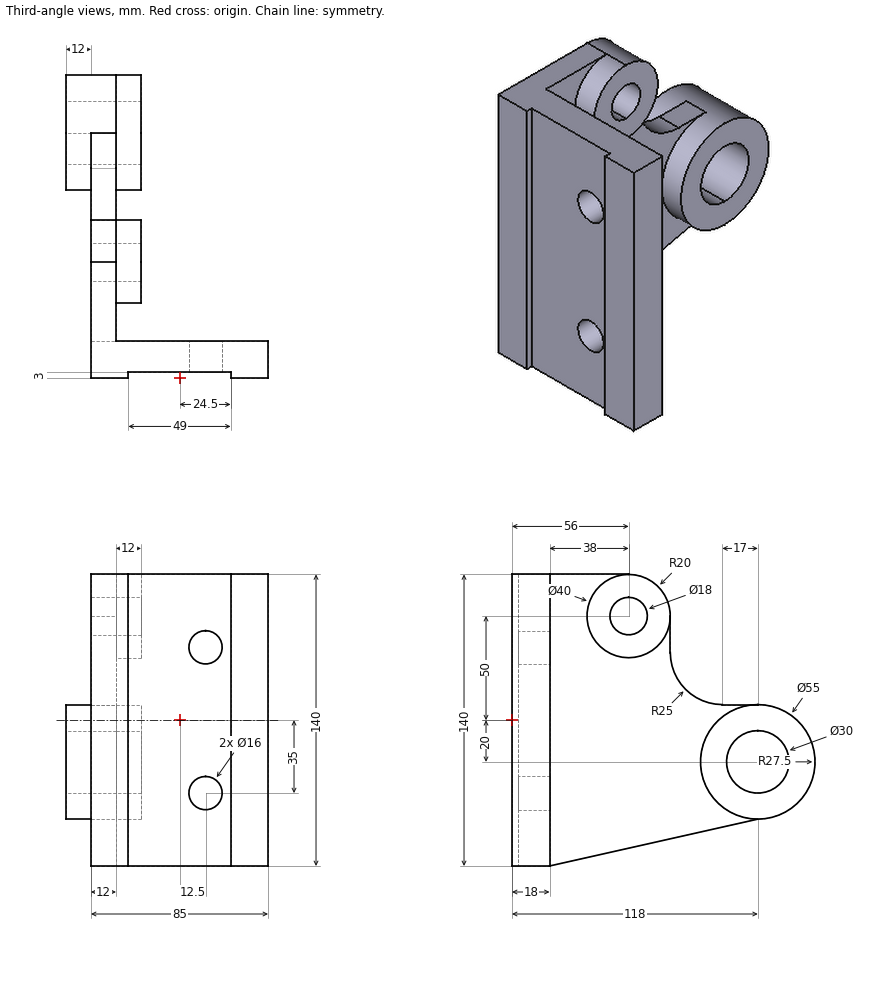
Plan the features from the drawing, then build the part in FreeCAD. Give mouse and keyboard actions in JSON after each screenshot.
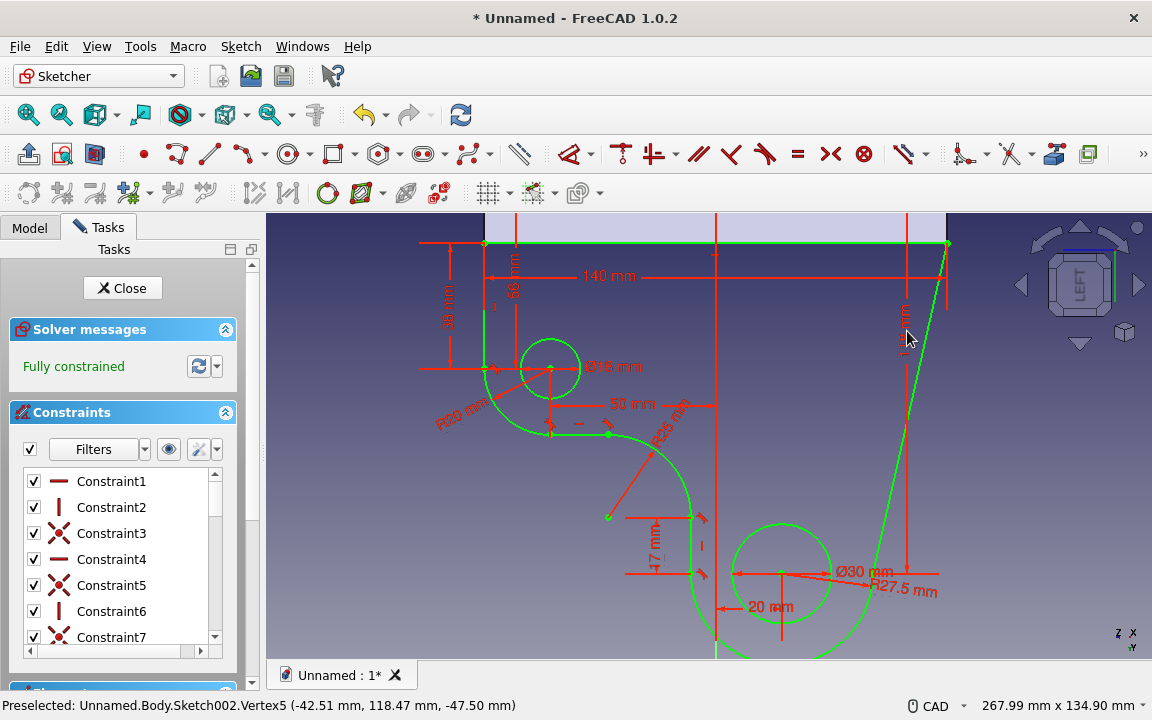
{"action": "left_click", "coordinate": [123, 288]}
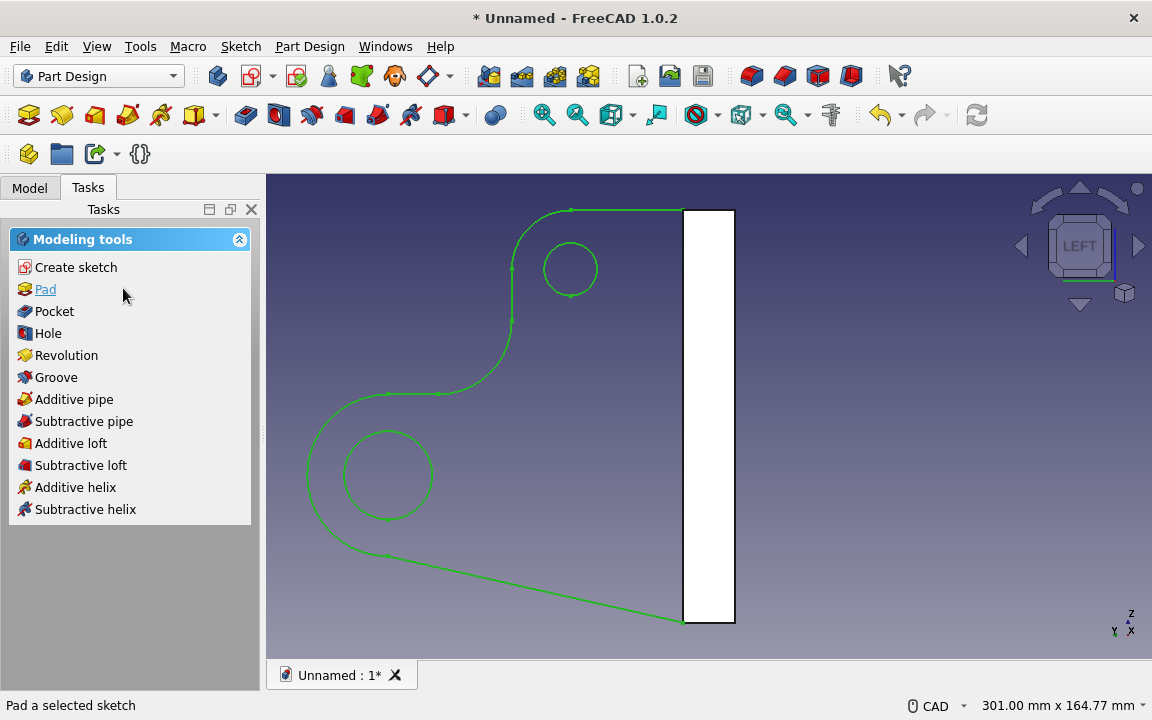
{"action": "left_click", "coordinate": [29, 116]}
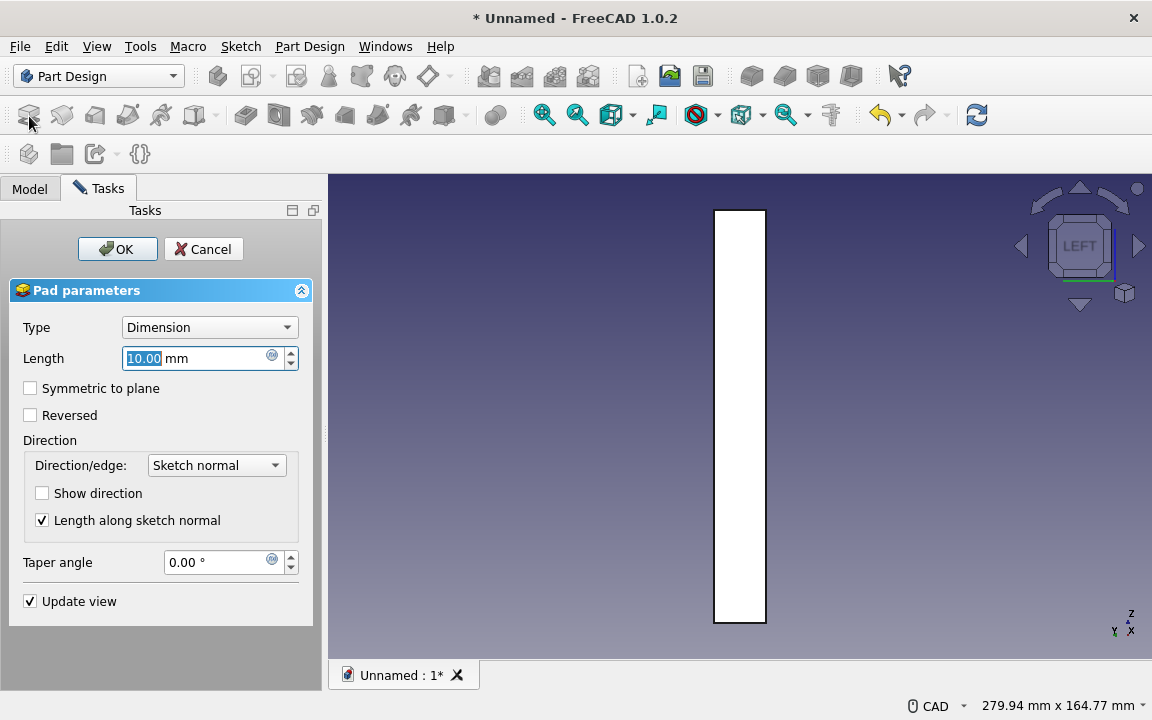
{"action": "type", "text": "12"}
{"action": "key", "text": "Tab"}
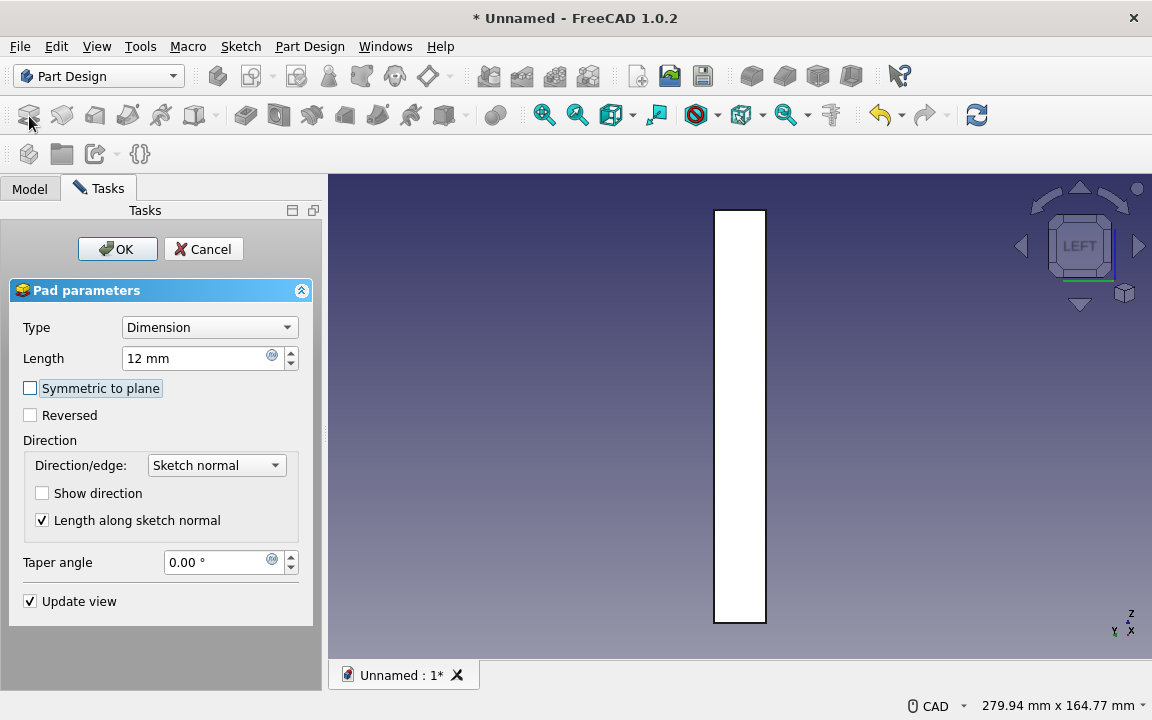
{"action": "left_click", "coordinate": [31, 415]}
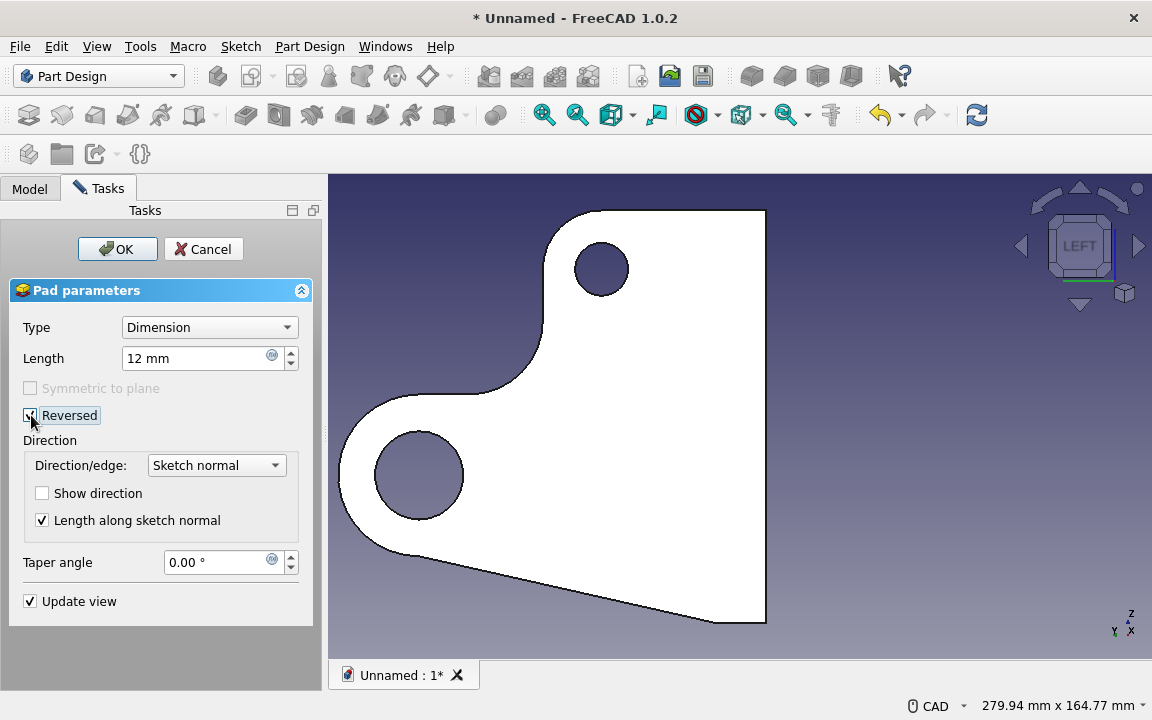
{"action": "left_click", "coordinate": [118, 249]}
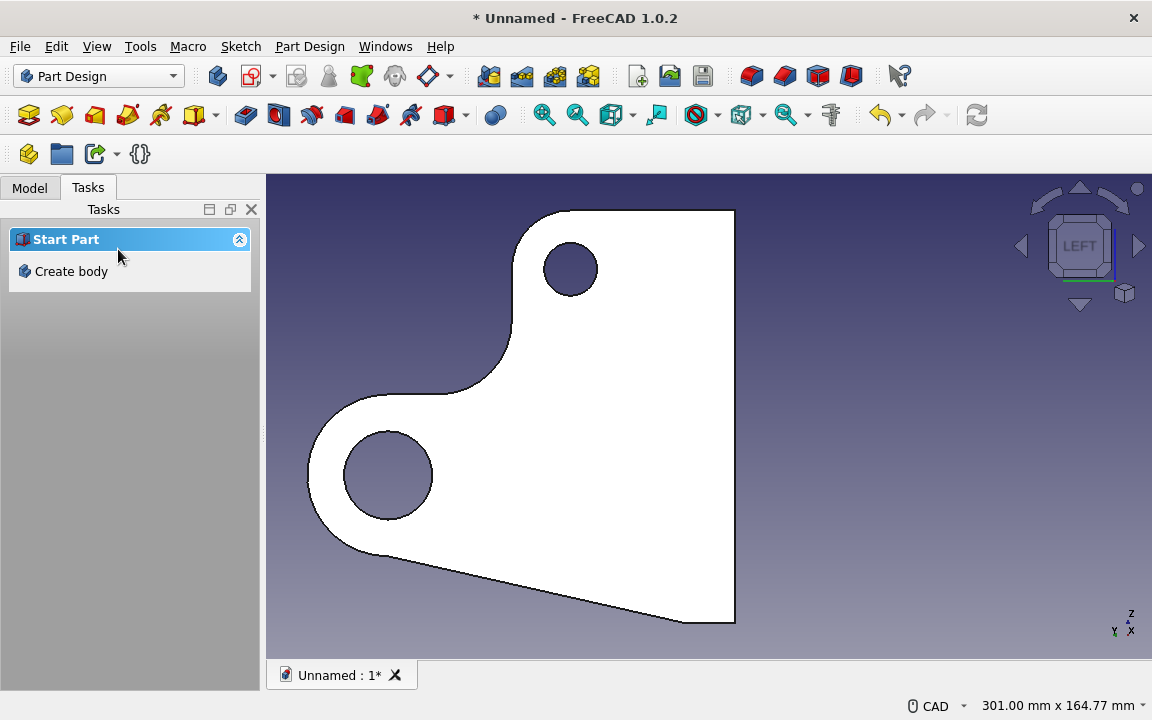
{"action": "key", "text": "0"}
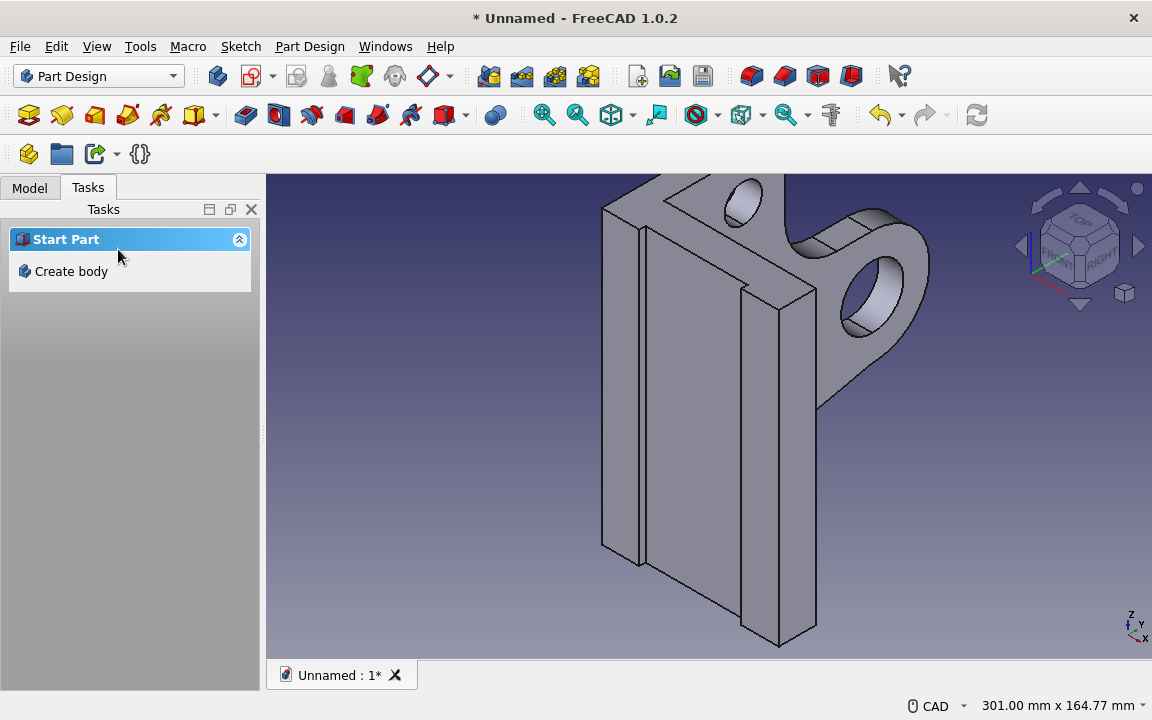
{"action": "key", "text": "v f"}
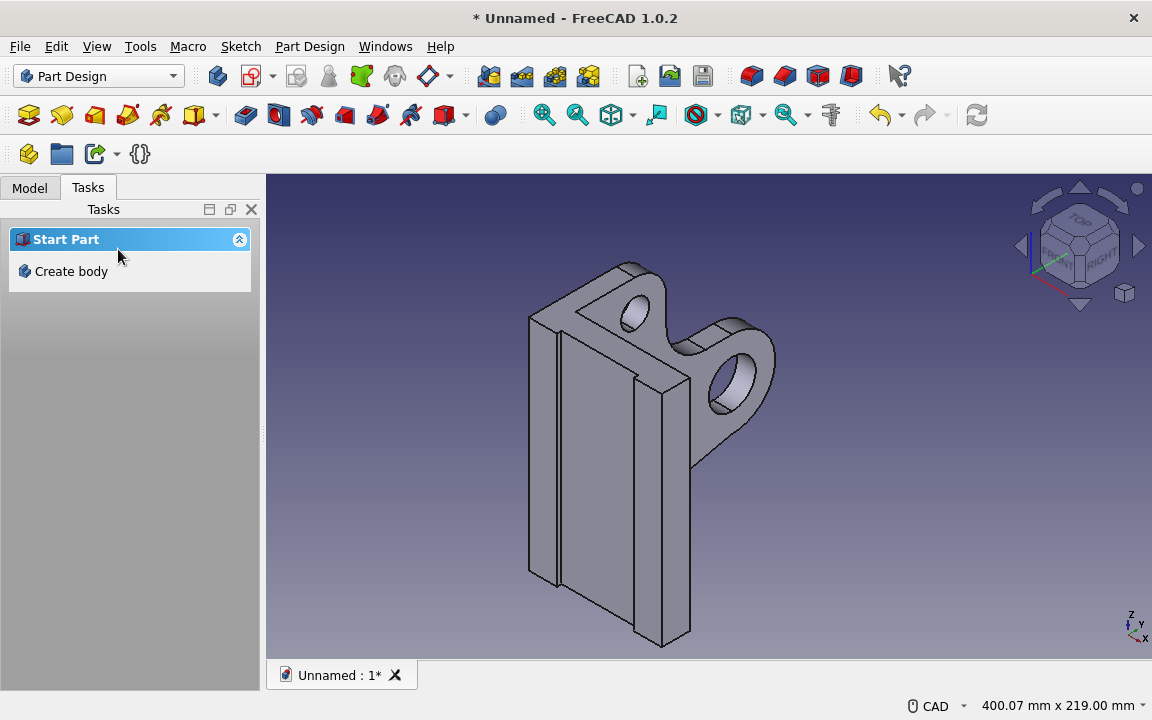
{"action": "key", "text": "3"}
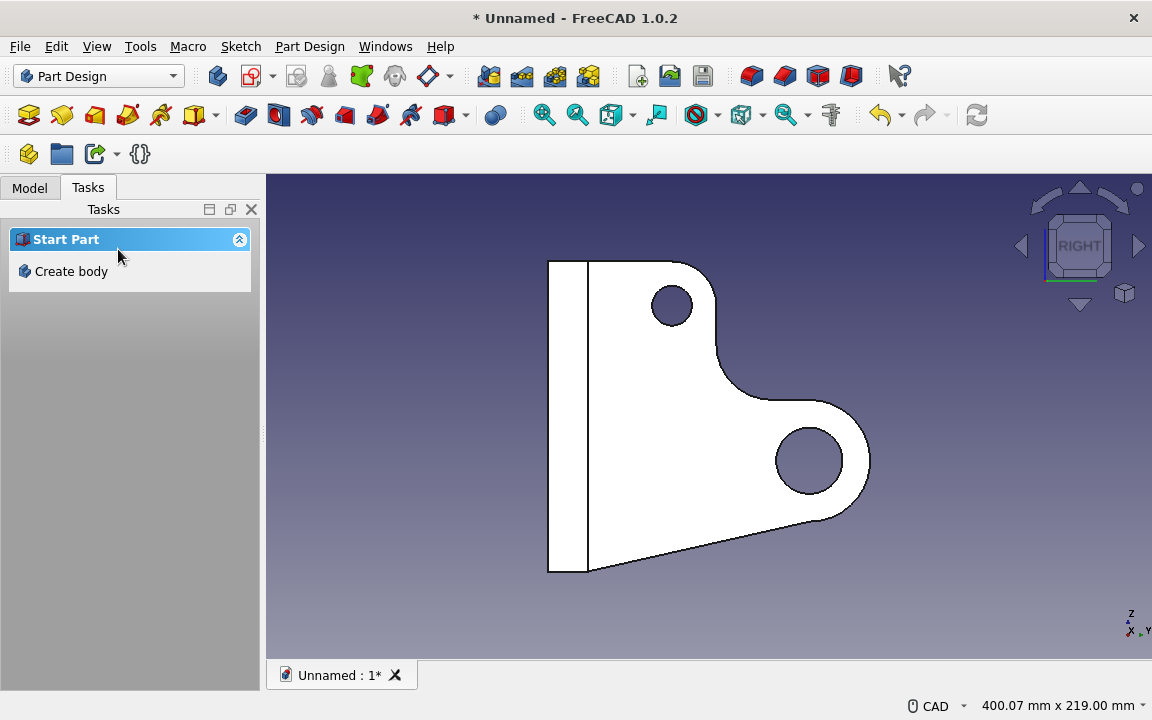
{"action": "left_click", "coordinate": [689, 460]}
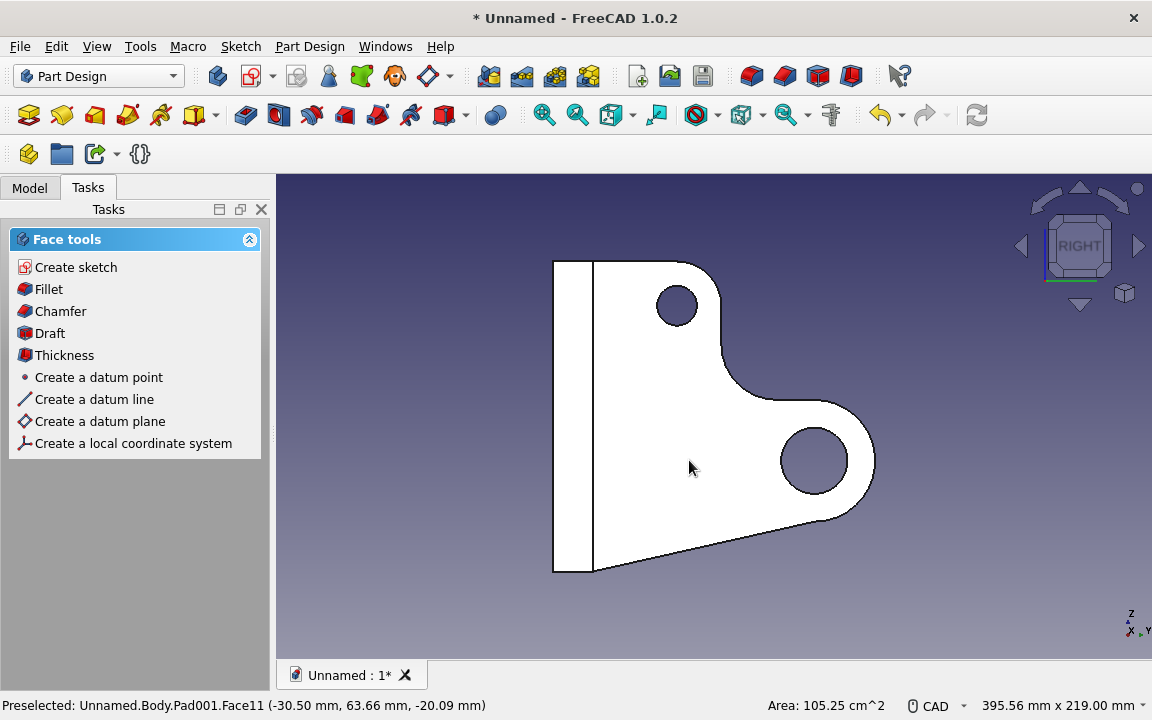
{"action": "left_click", "coordinate": [250, 76]}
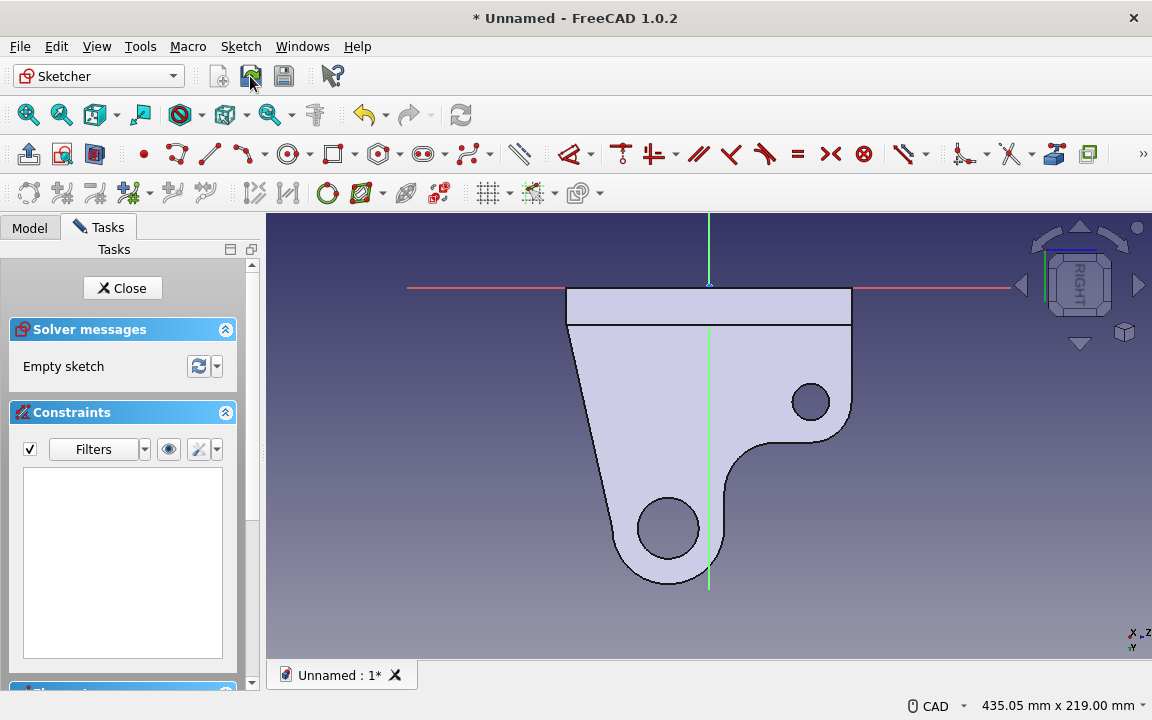
{"action": "scroll", "coordinate": [950, 279], "scroll_direction": "up", "scroll_amount": 3}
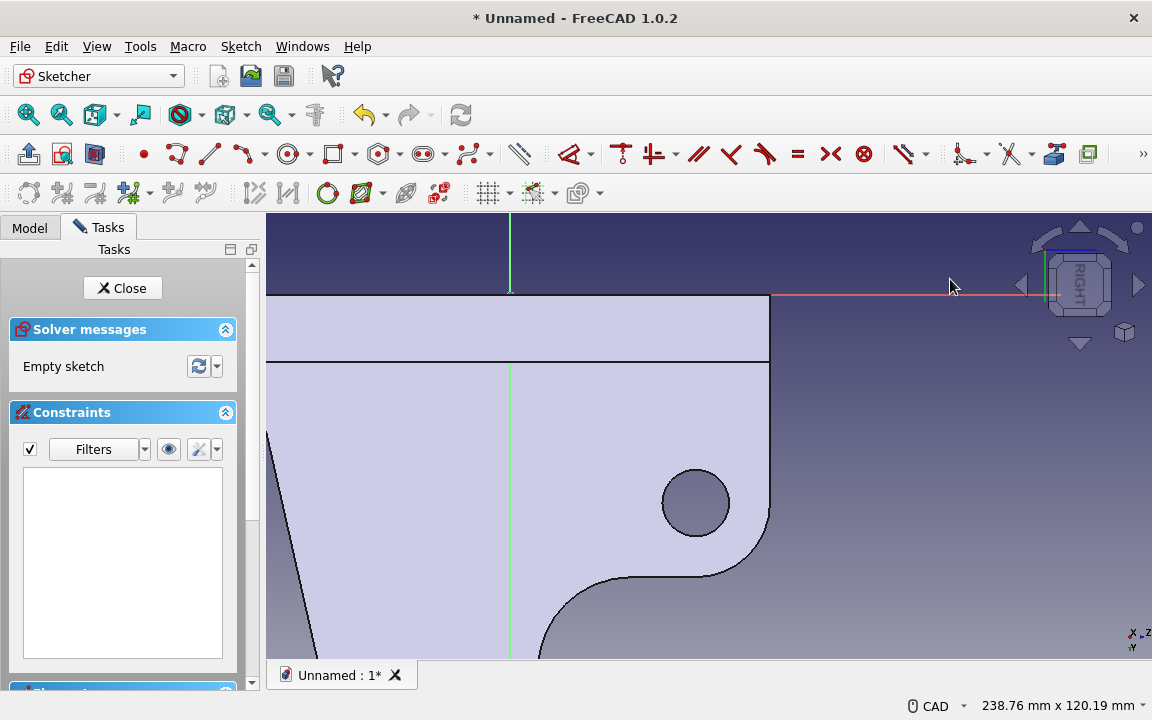
{"action": "left_click", "coordinate": [288, 154]}